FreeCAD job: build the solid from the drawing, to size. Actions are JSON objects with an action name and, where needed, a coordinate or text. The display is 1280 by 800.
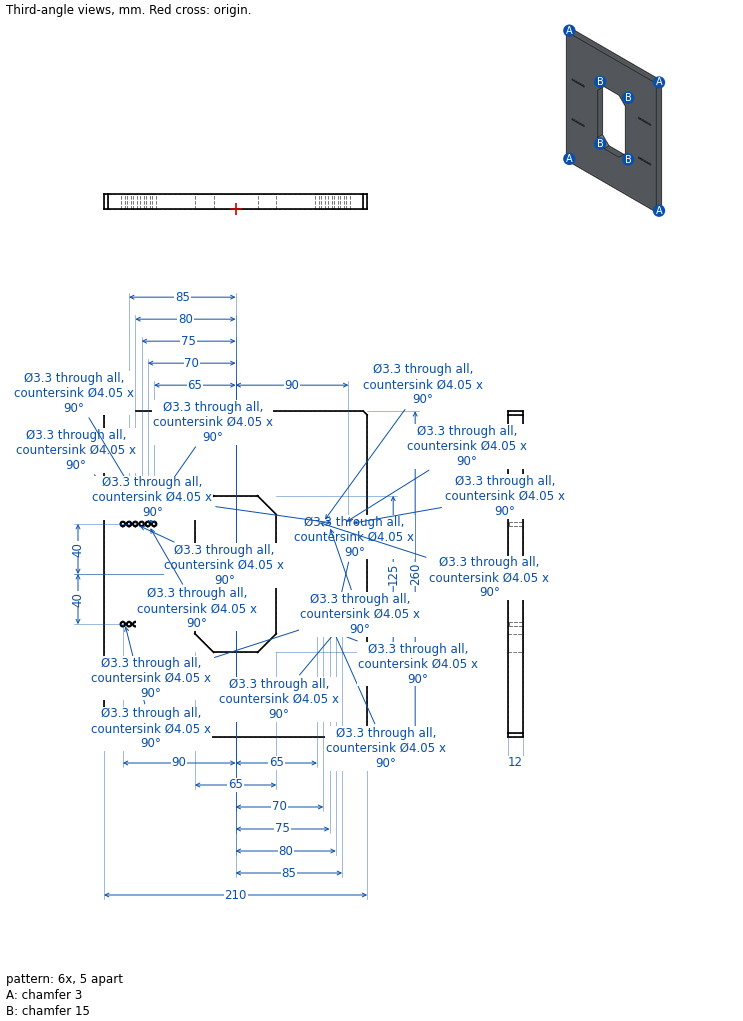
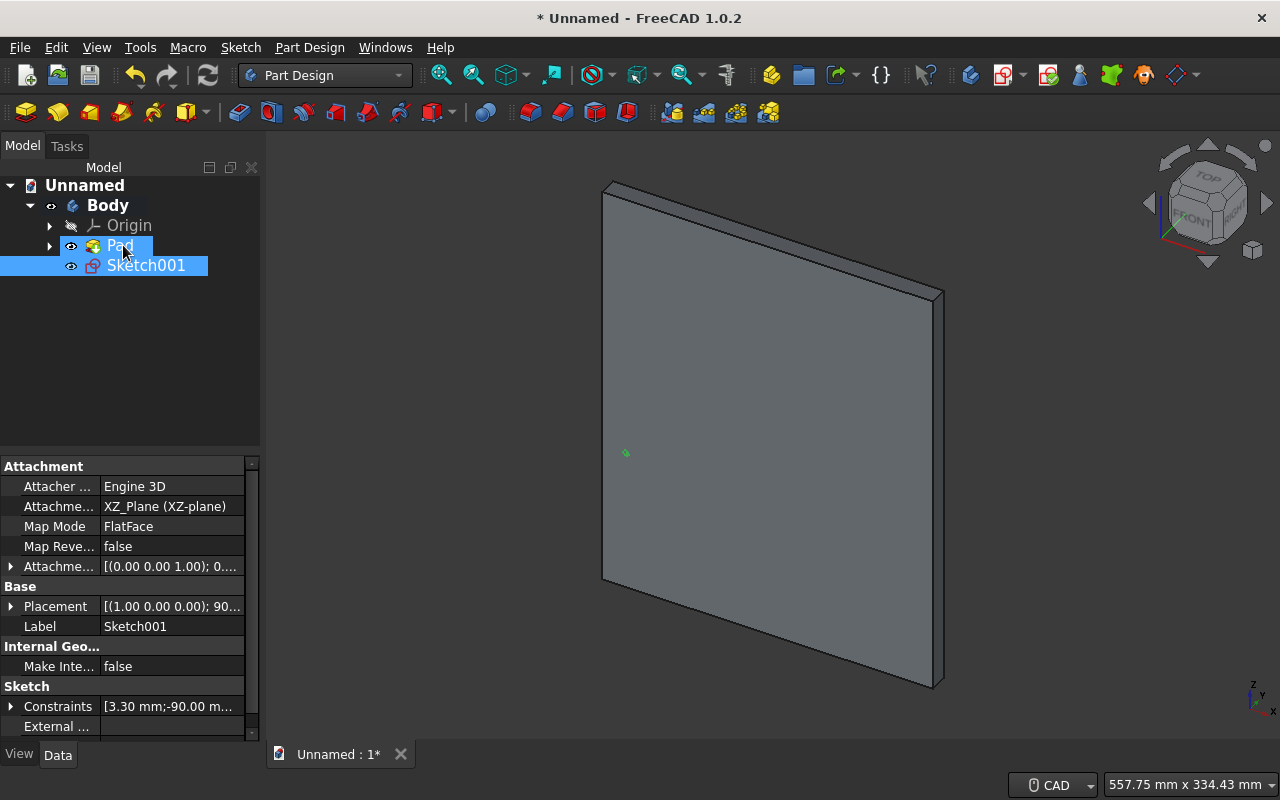
{"action": "left_click", "coordinate": [272, 112]}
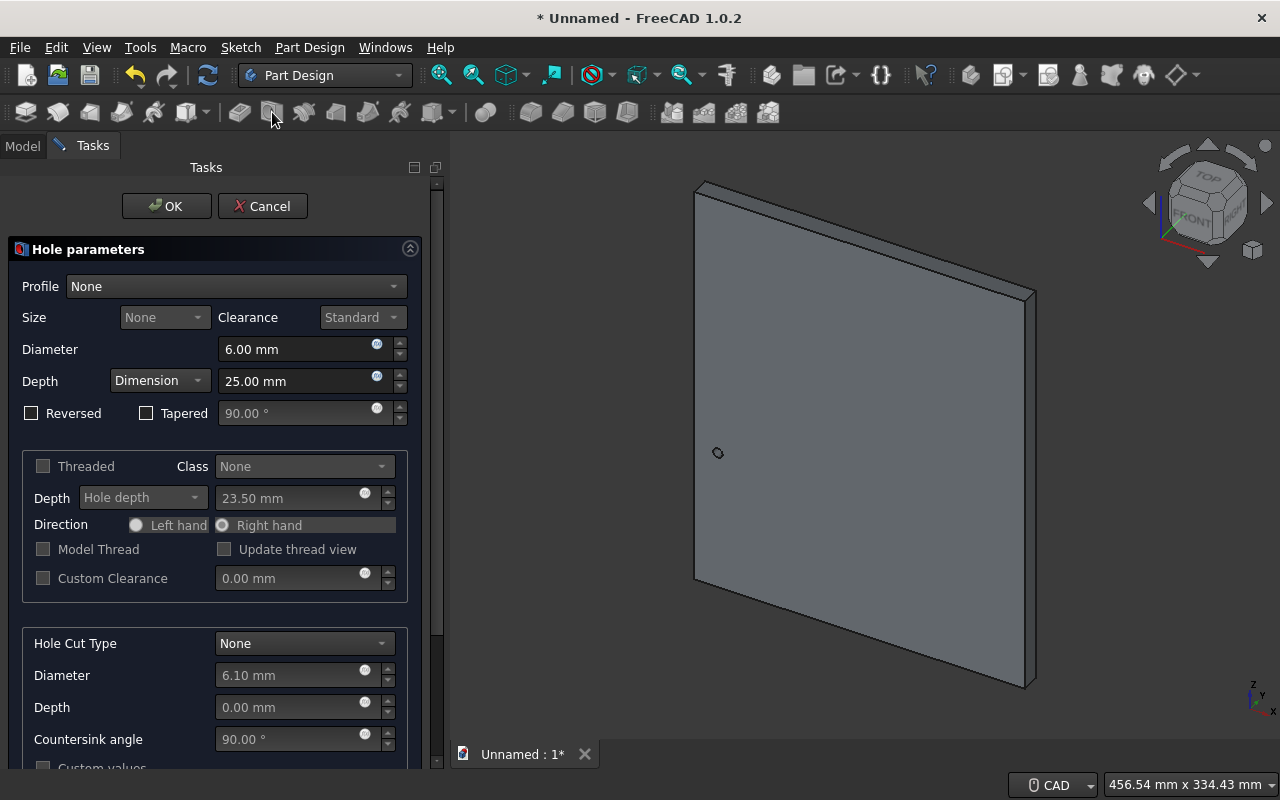
{"action": "triple_click", "coordinate": [305, 349]}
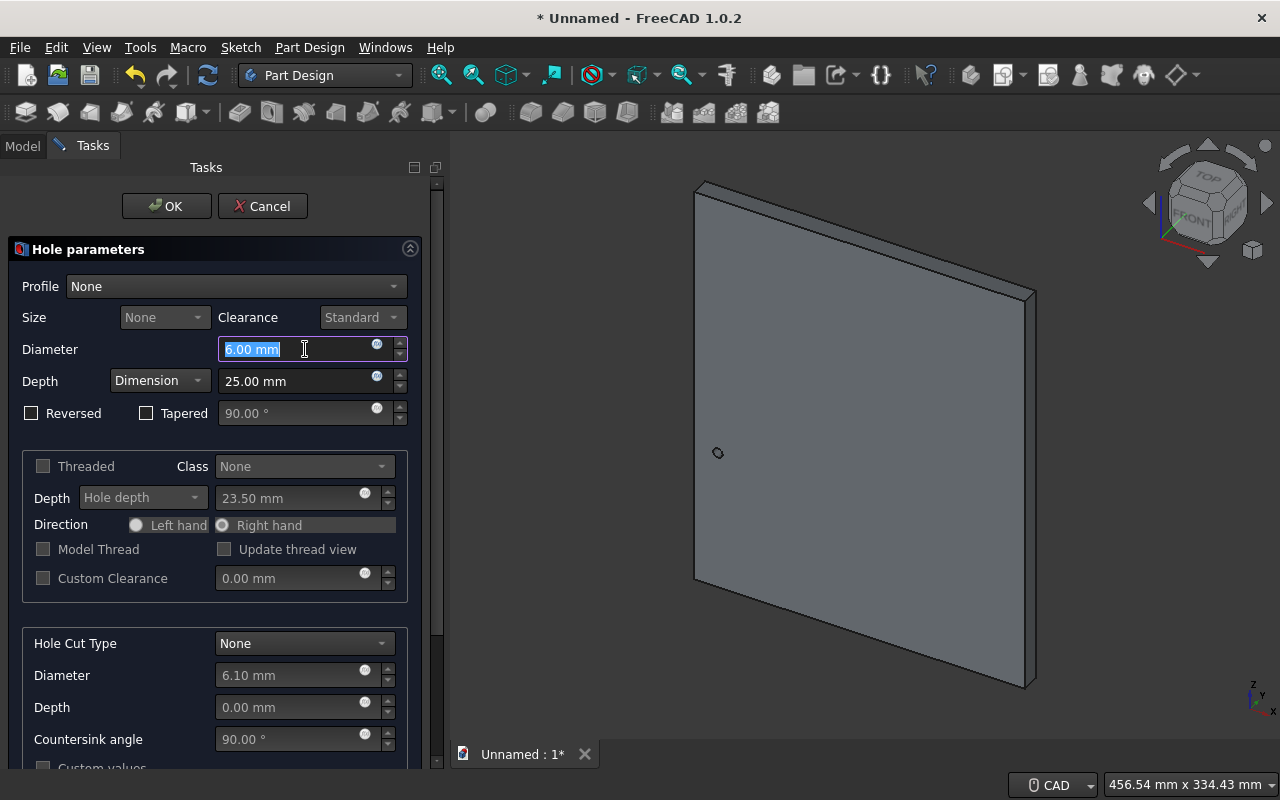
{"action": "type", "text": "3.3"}
{"action": "key", "text": "Tab"}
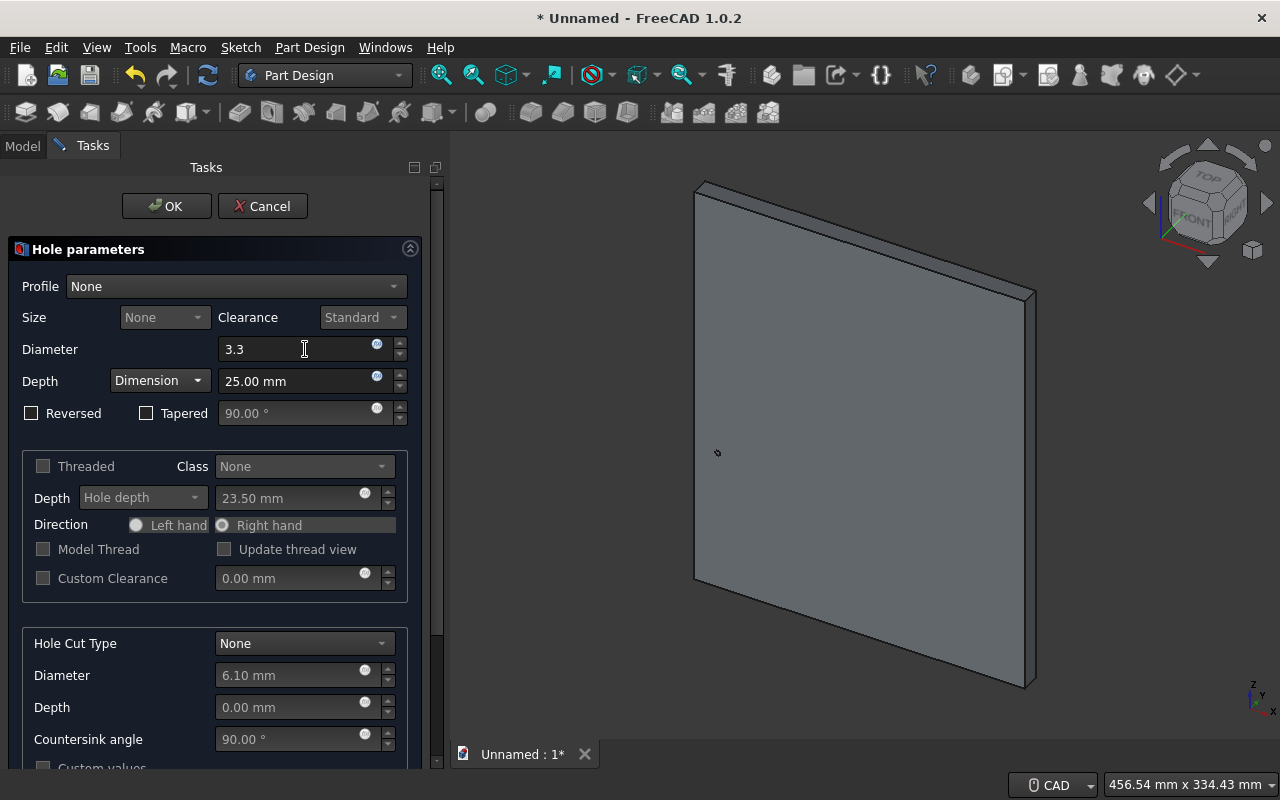
{"action": "left_click", "coordinate": [161, 380]}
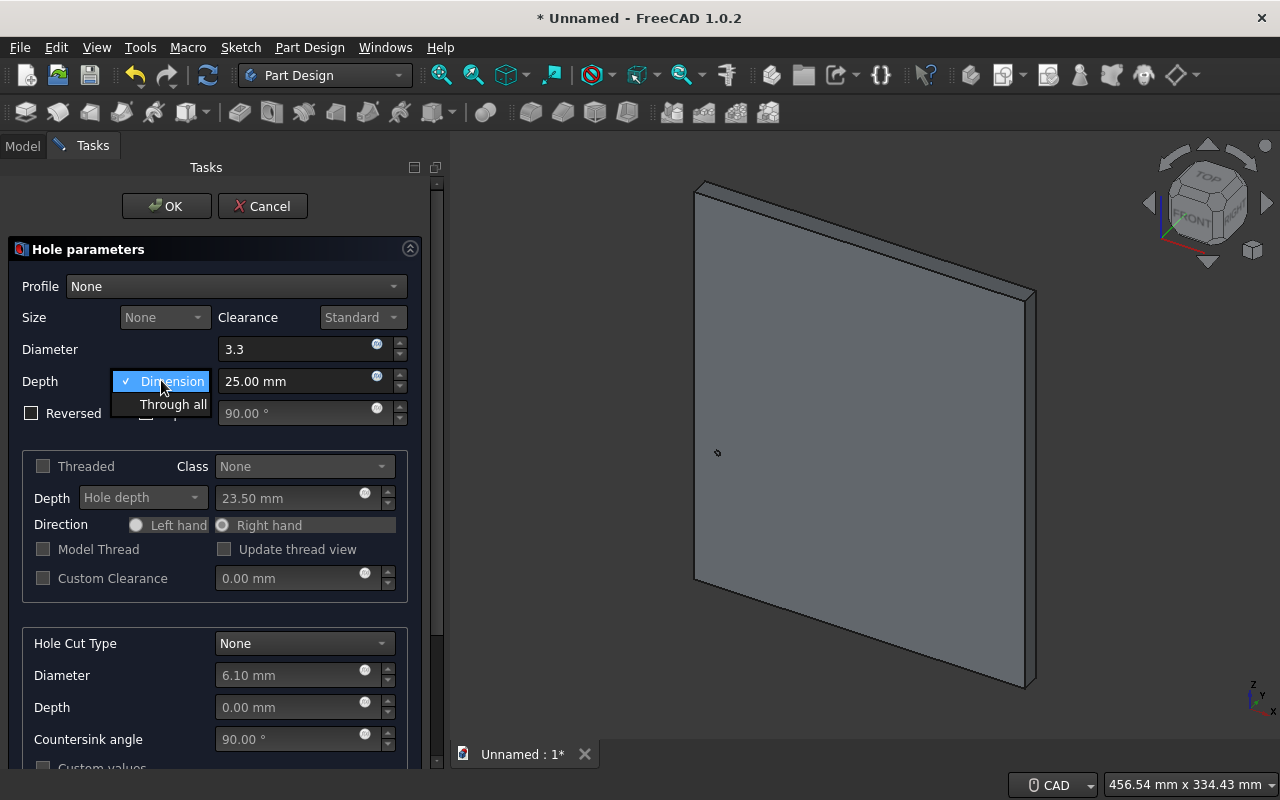
{"action": "left_click", "coordinate": [160, 404]}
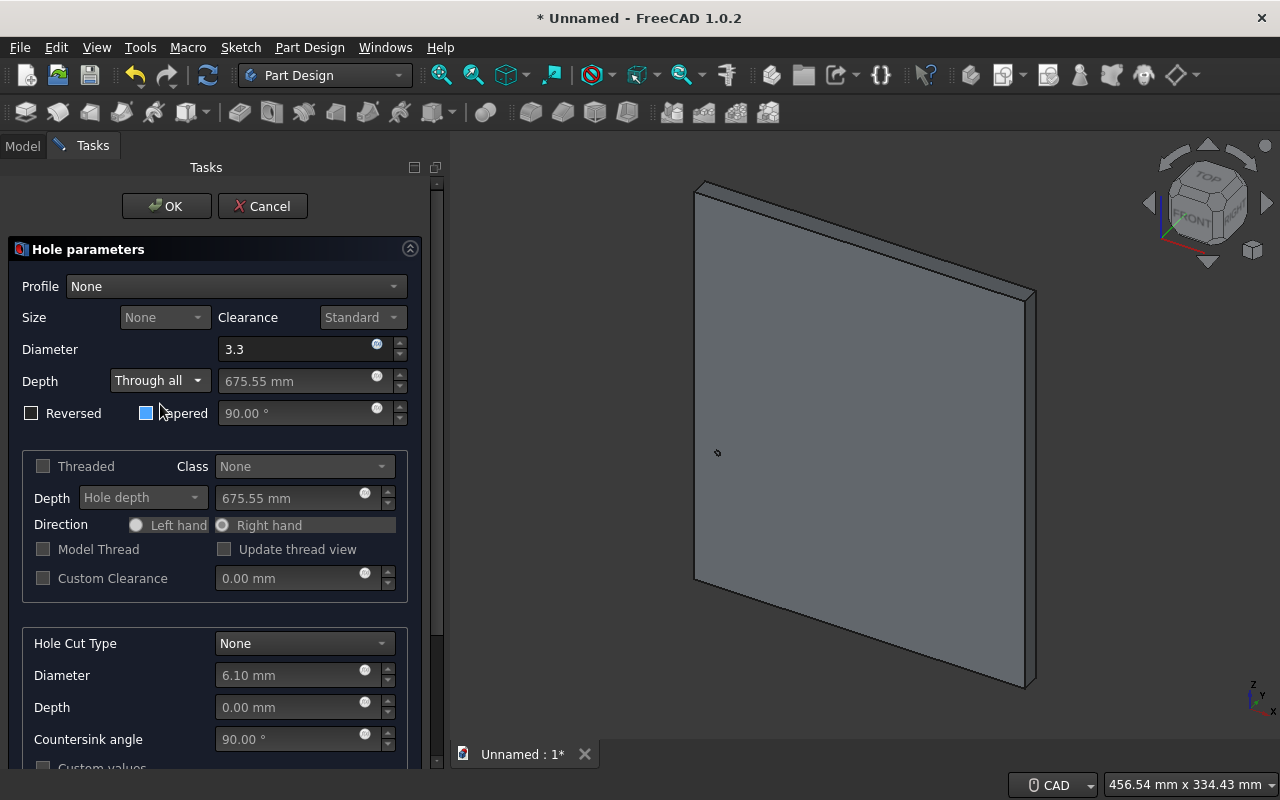
{"action": "left_click", "coordinate": [306, 644]}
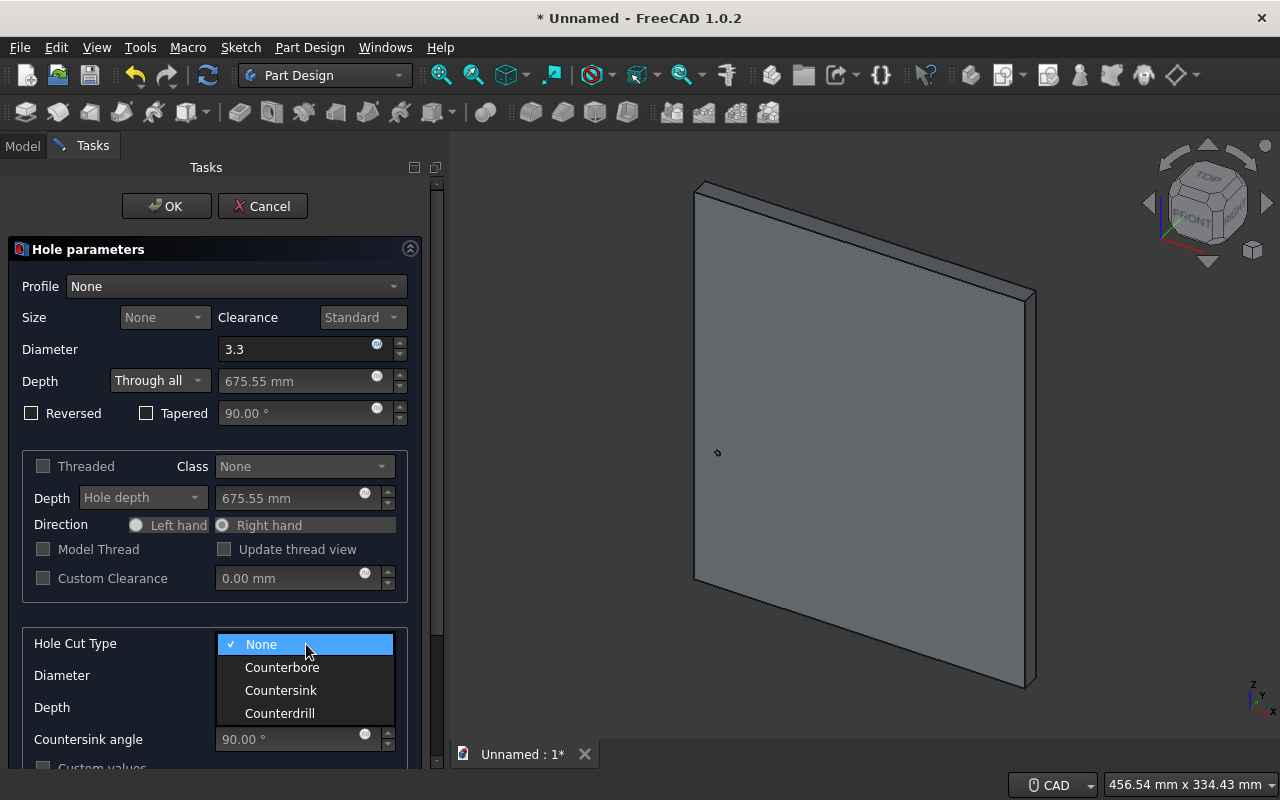
{"action": "left_click", "coordinate": [304, 690]}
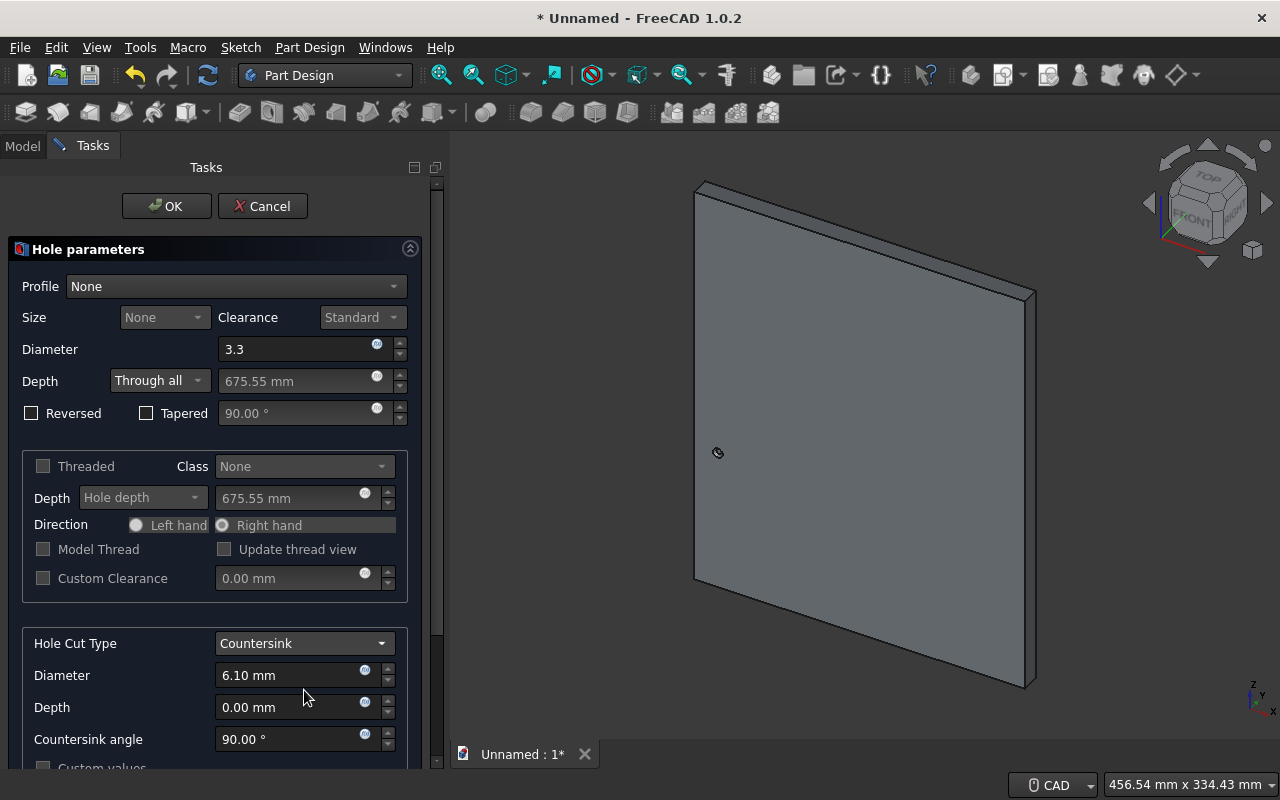
{"action": "triple_click", "coordinate": [298, 675]}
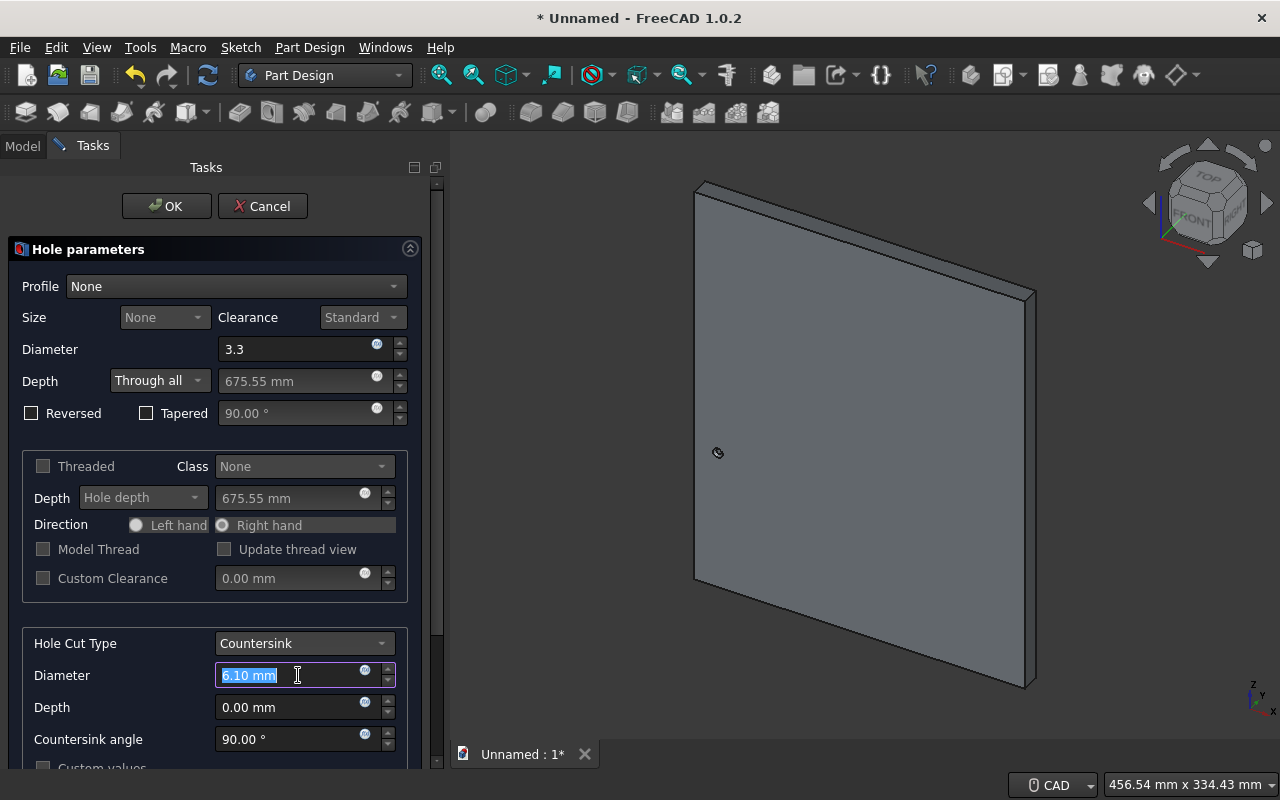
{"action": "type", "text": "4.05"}
{"action": "key", "text": "Tab"}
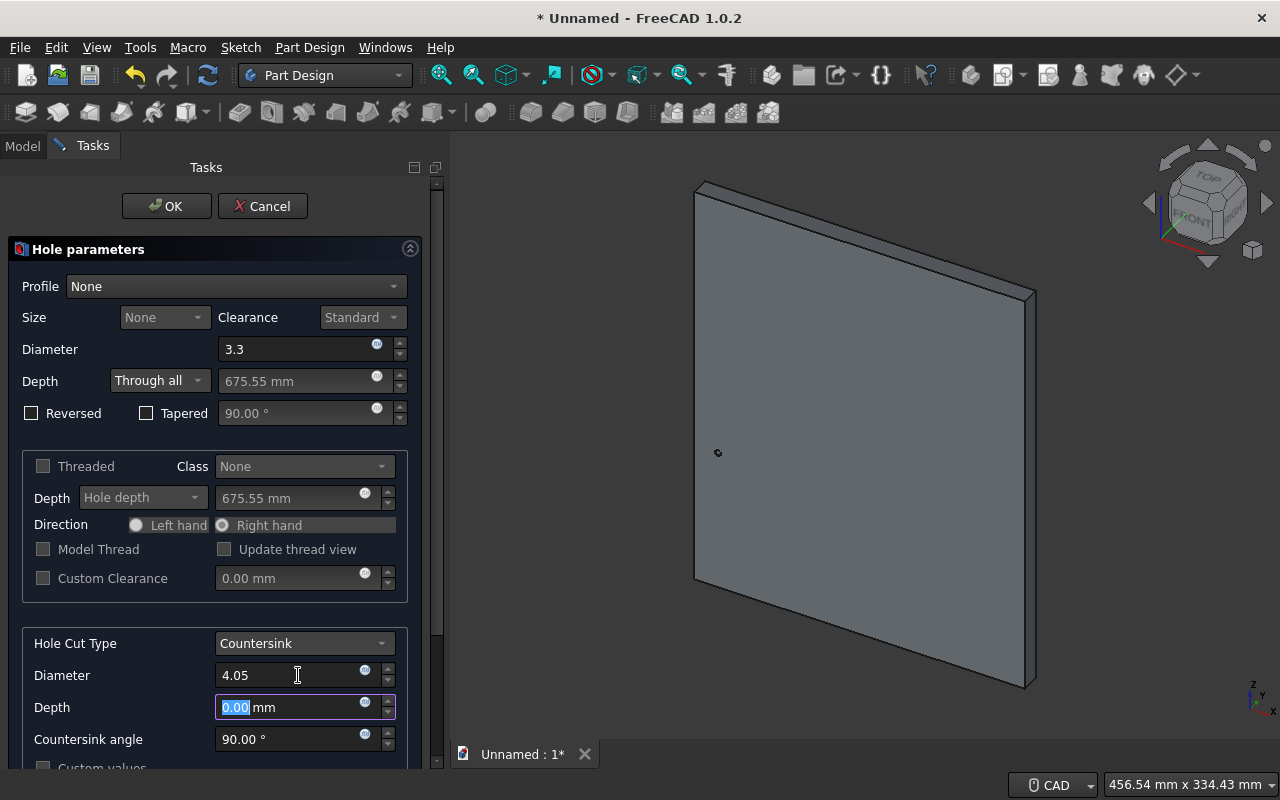
{"action": "left_click", "coordinate": [167, 206]}